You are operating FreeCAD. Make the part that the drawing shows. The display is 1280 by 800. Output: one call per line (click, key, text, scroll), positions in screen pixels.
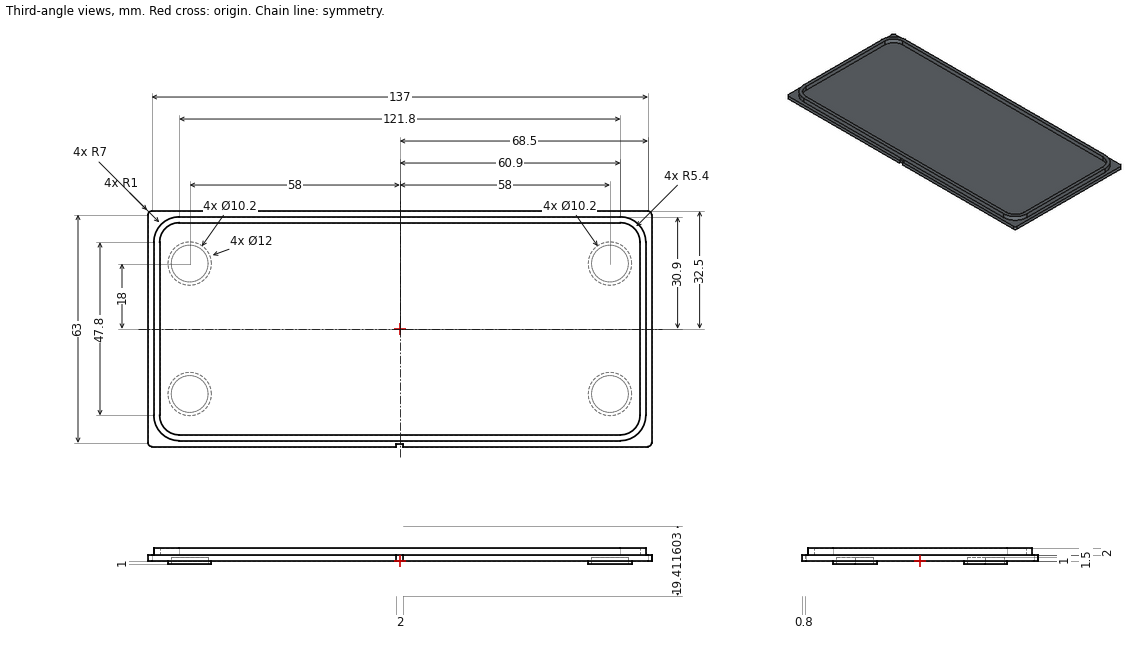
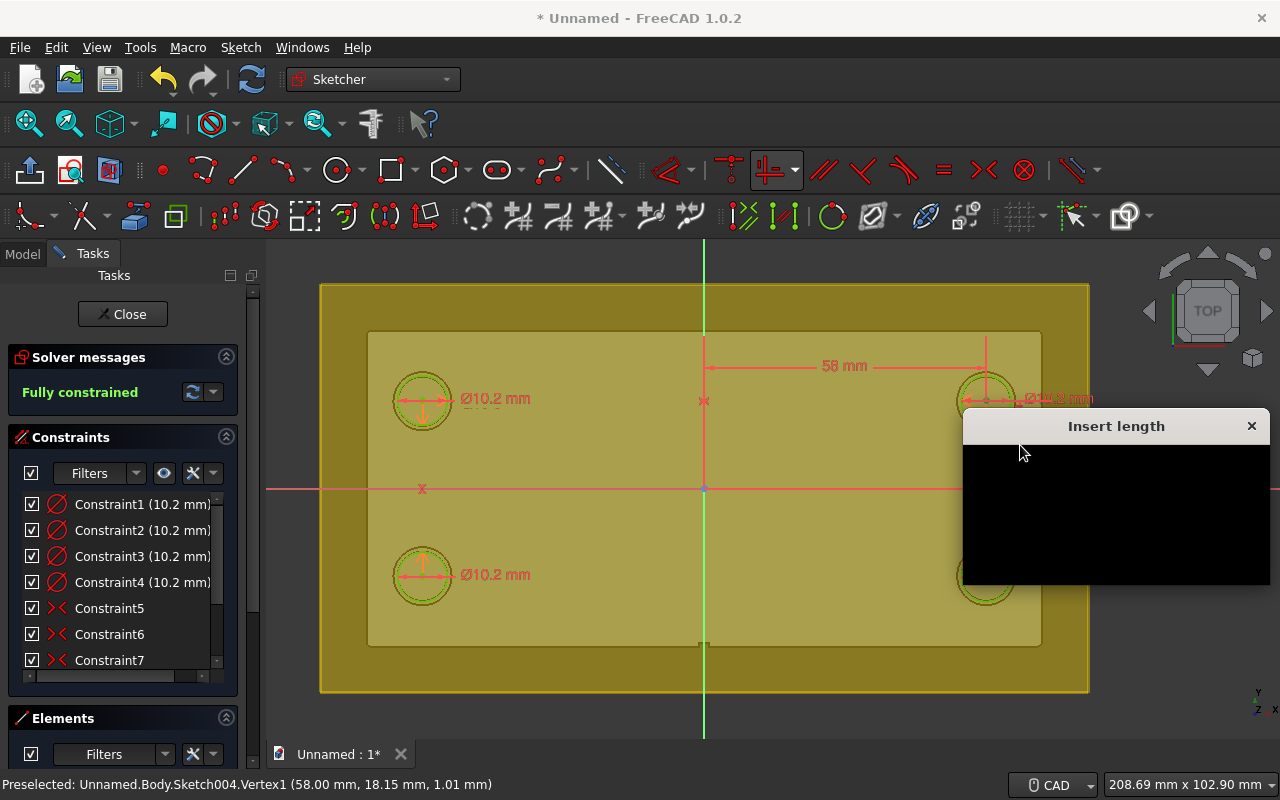
text(18)
key(Return)
key(Escape)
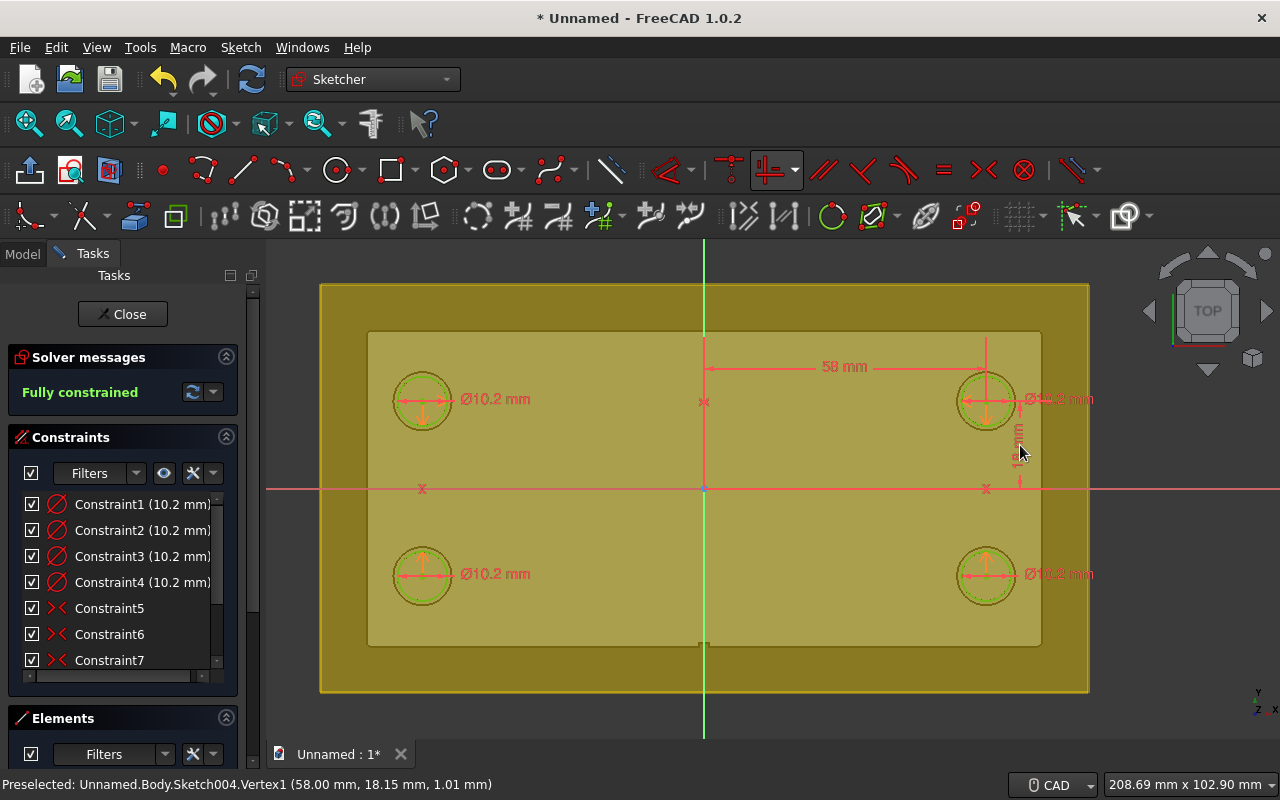
click(123, 314)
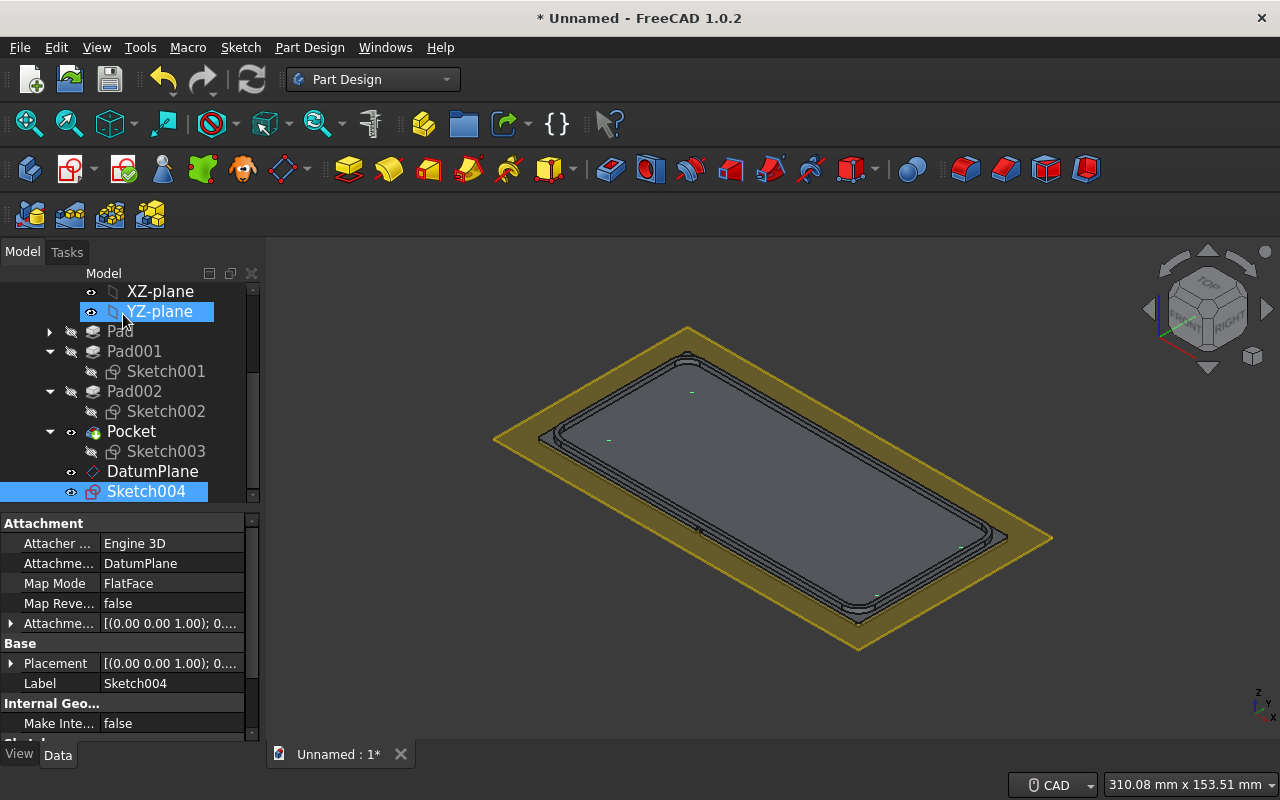
click(612, 170)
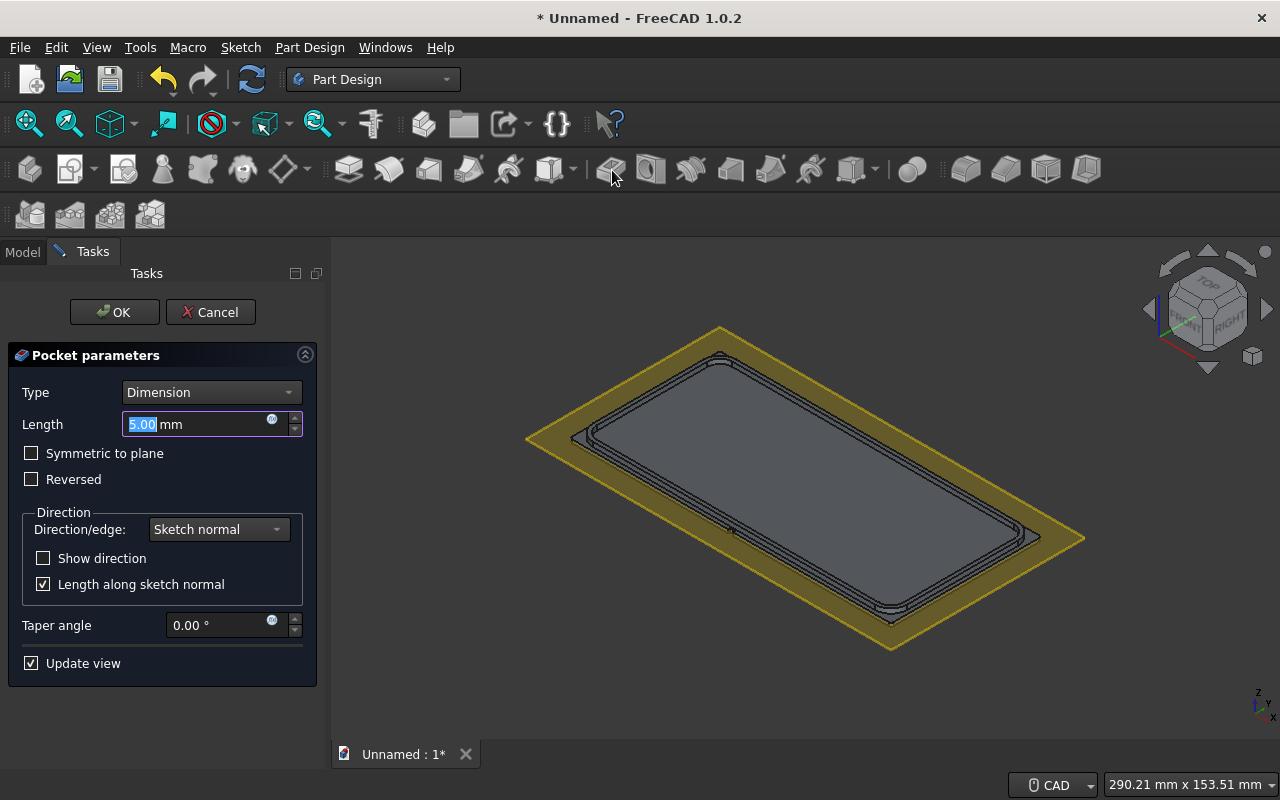
text(1)
key(Tab)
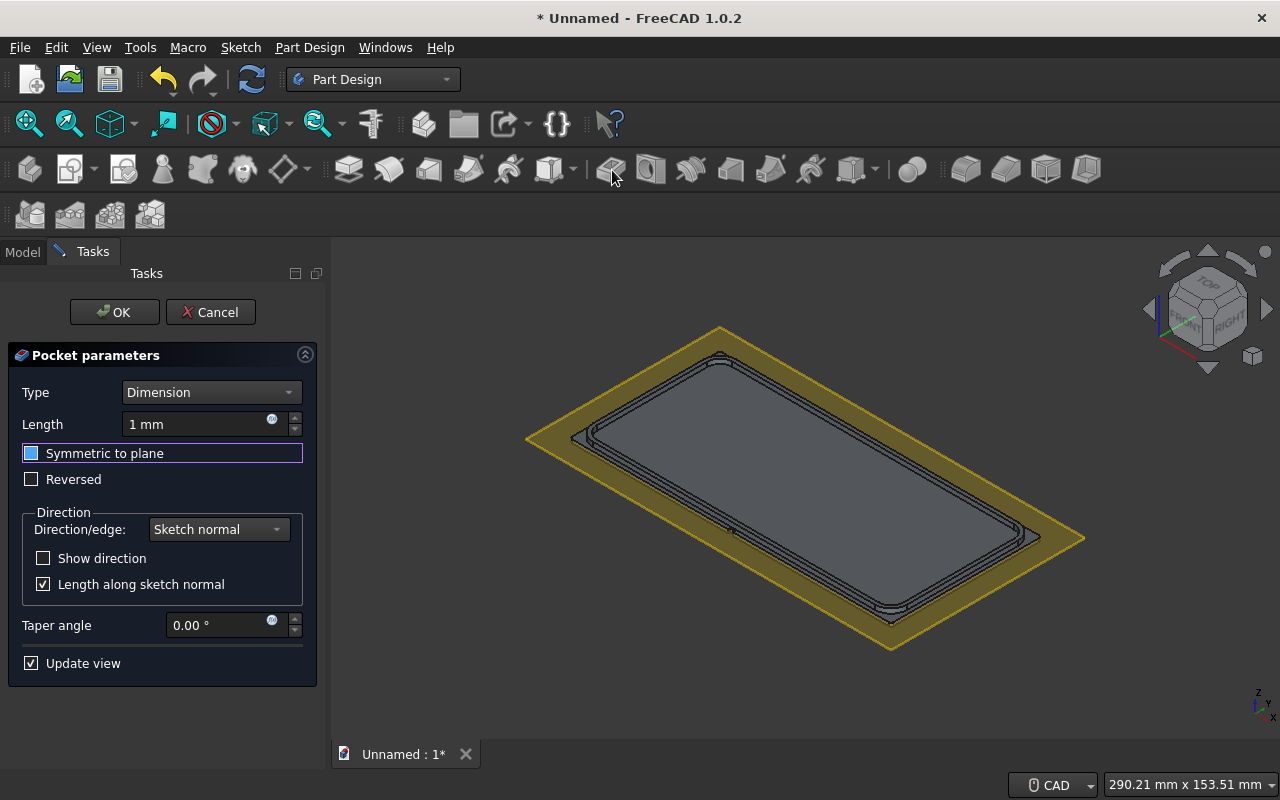
click(115, 312)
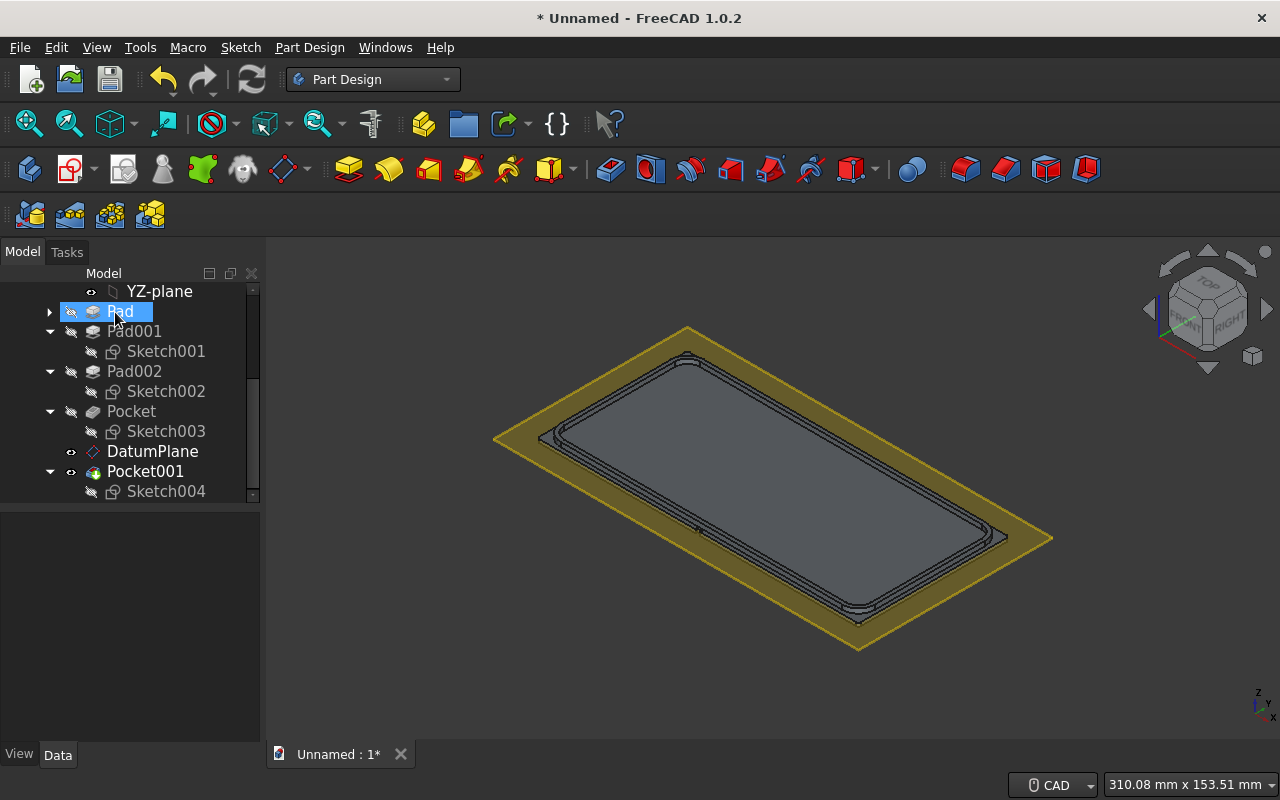
click(116, 452)
key(space)